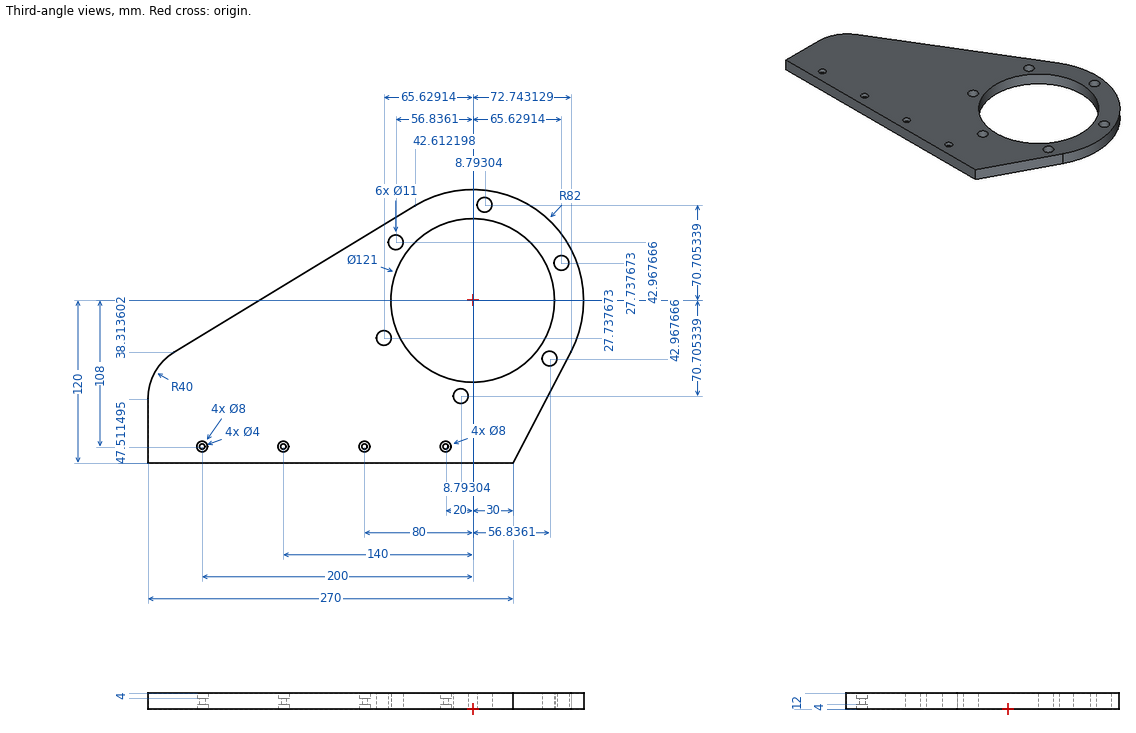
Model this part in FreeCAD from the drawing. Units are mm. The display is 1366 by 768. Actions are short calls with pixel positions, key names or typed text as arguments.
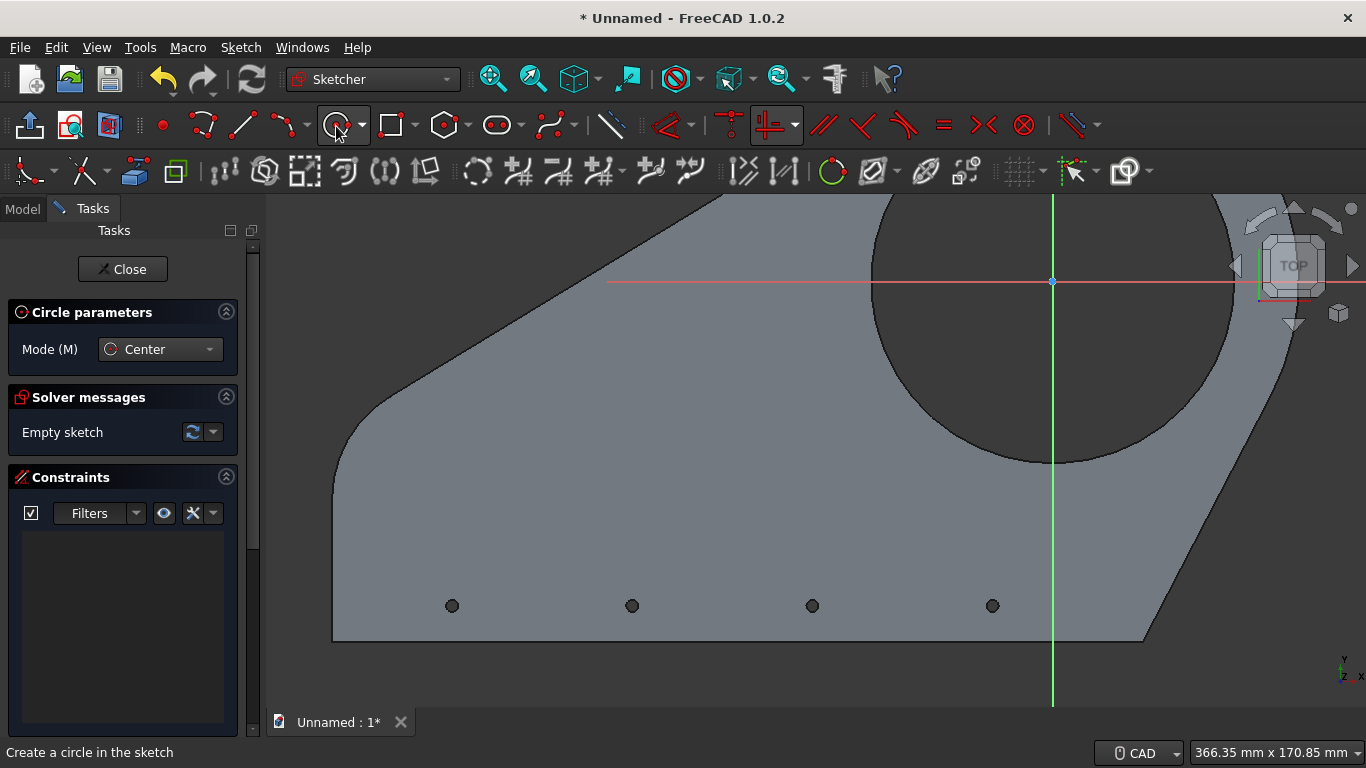
scroll(452, 606, up, 4)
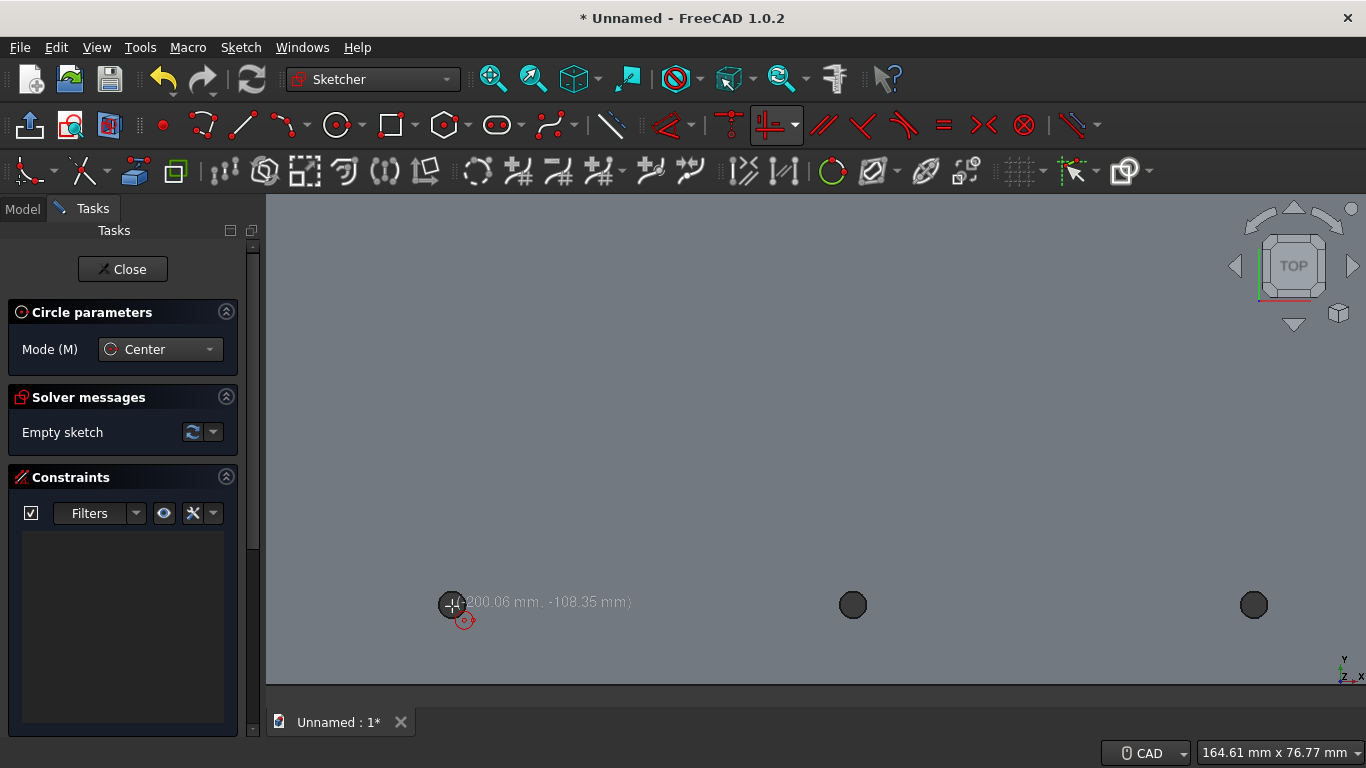
click(452, 605)
click(471, 586)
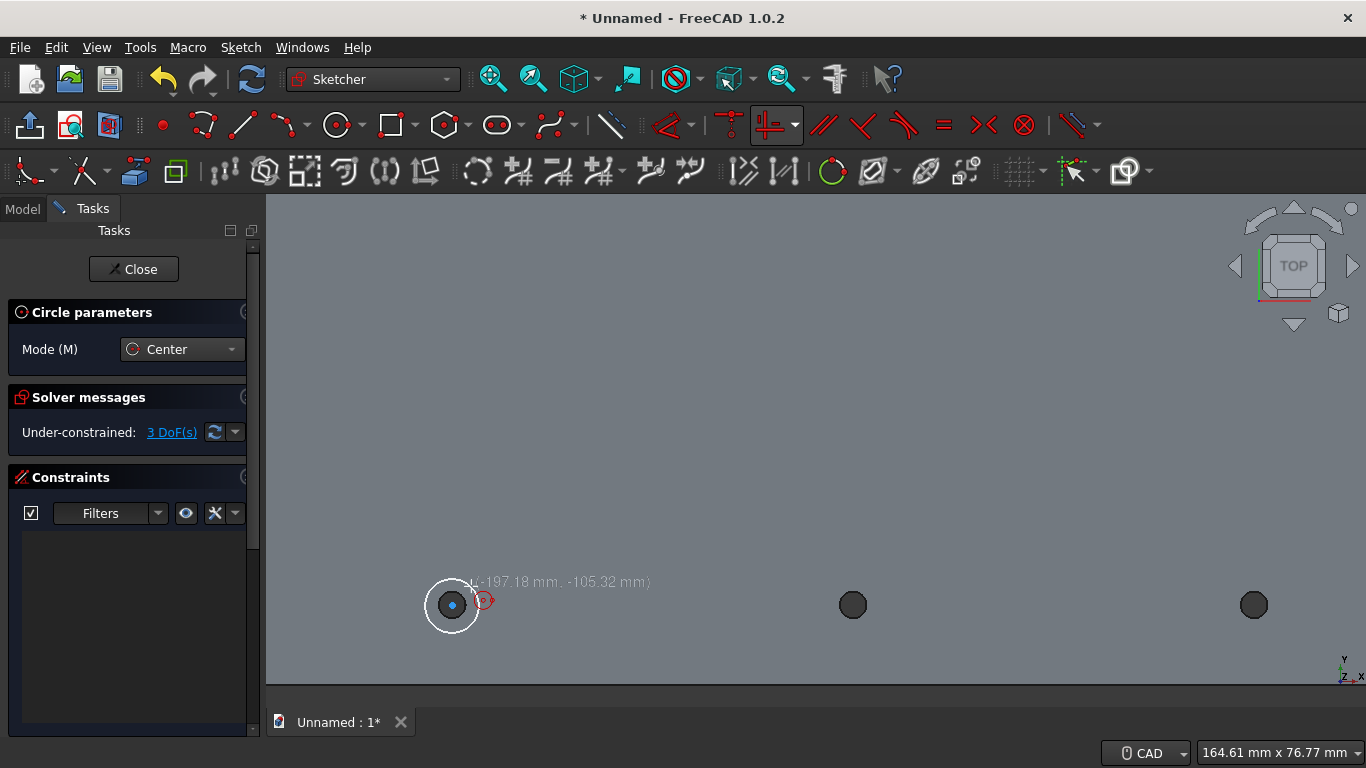
click(853, 605)
click(872, 586)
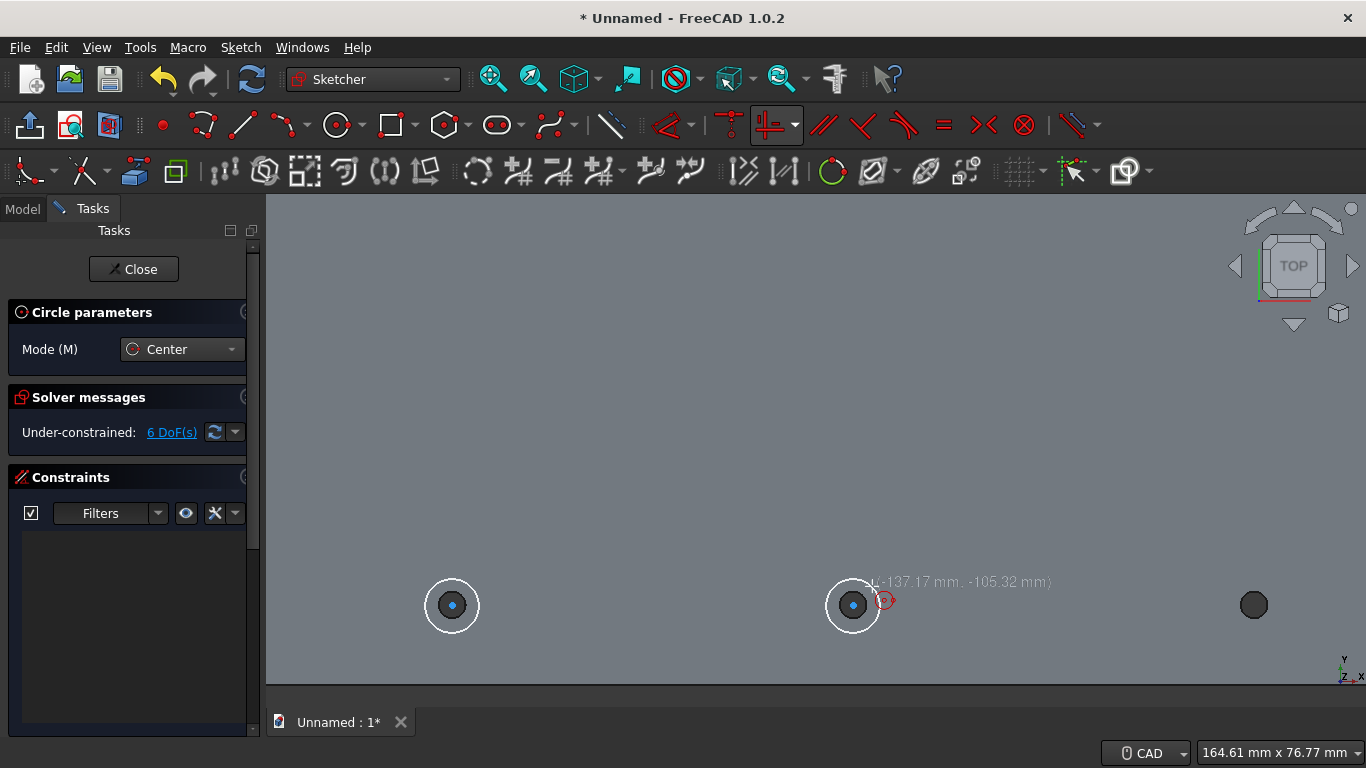
scroll(454, 608, down, 4)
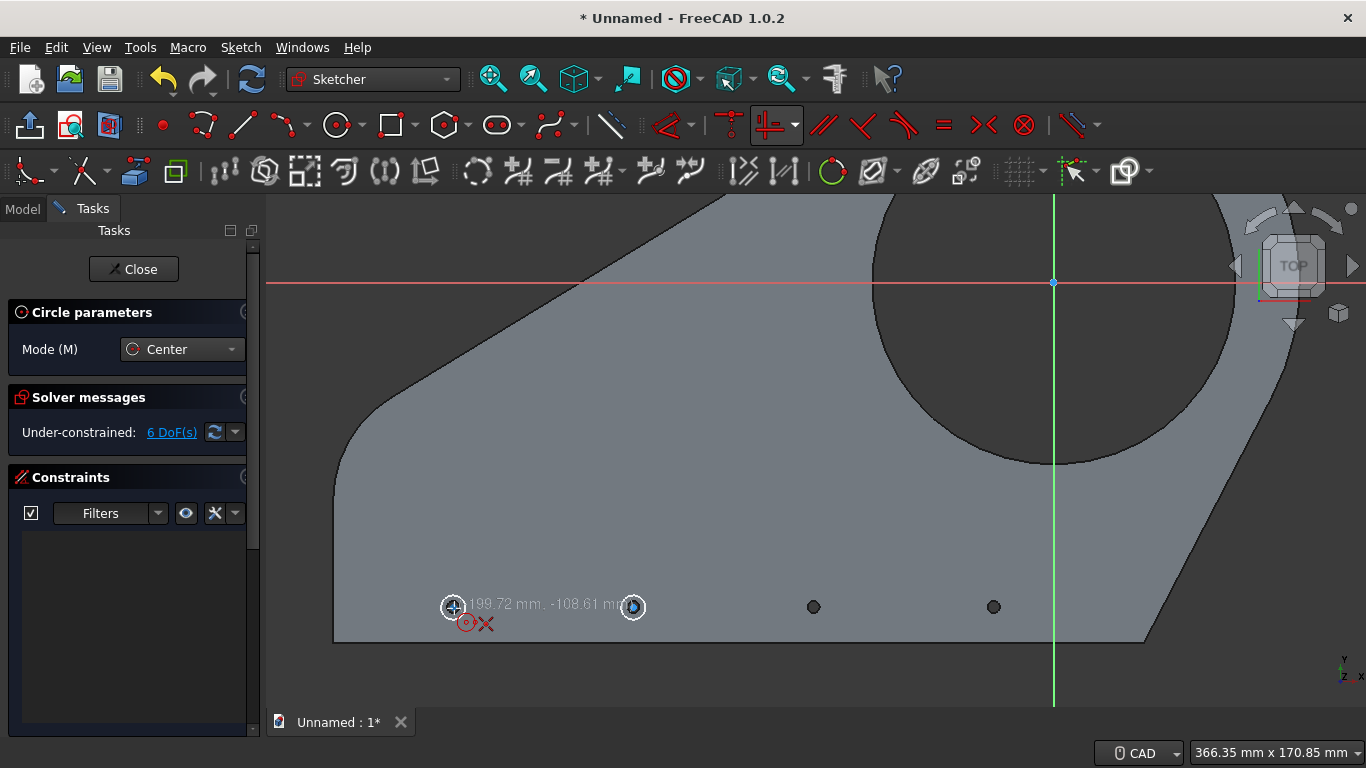
scroll(814, 607, up, 4)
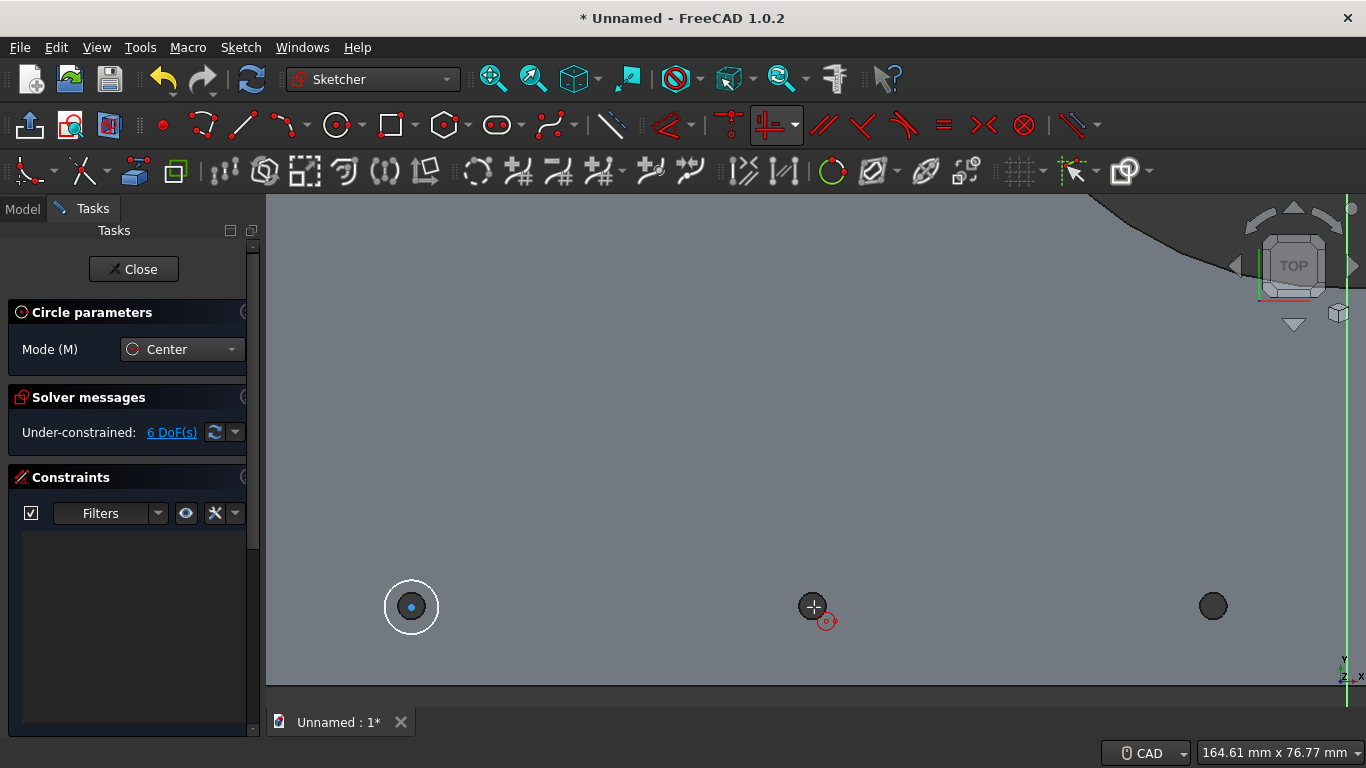
click(812, 606)
click(831, 587)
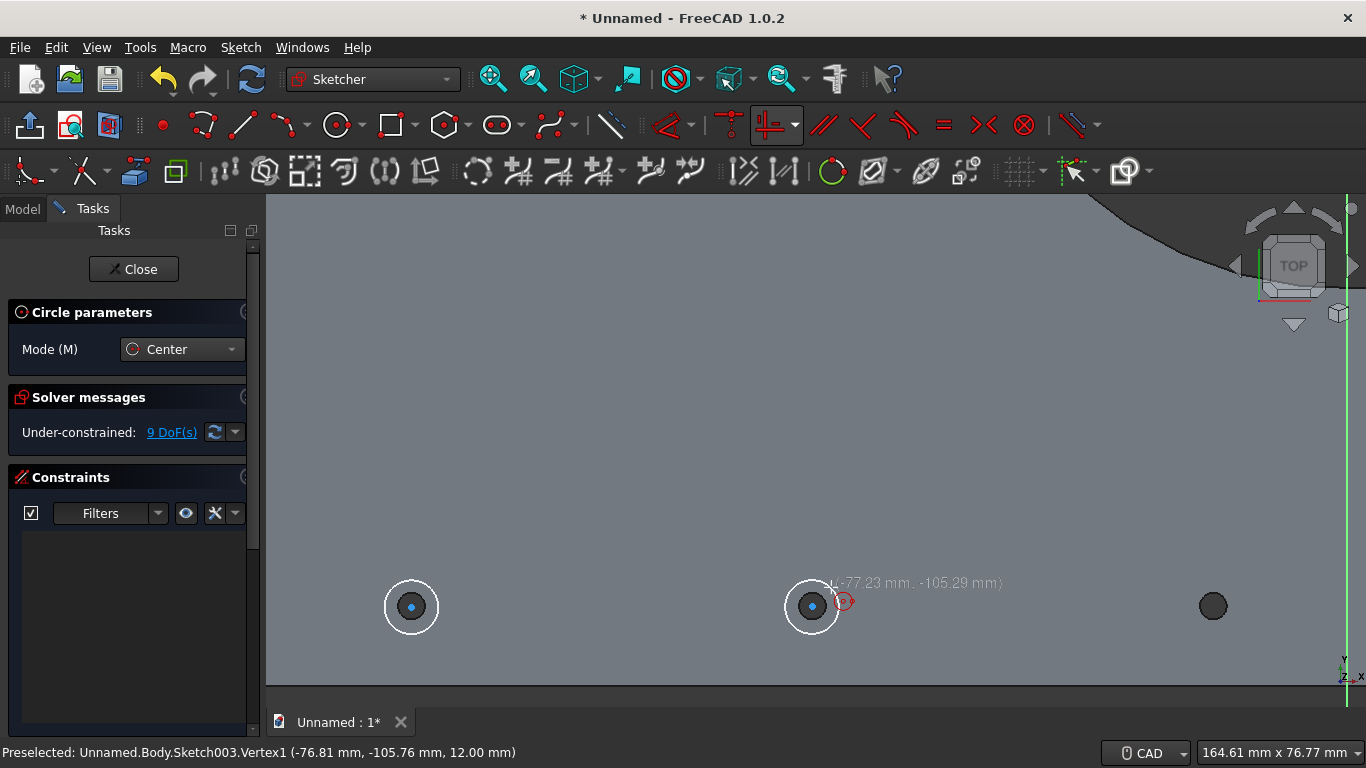
scroll(814, 607, down, 4)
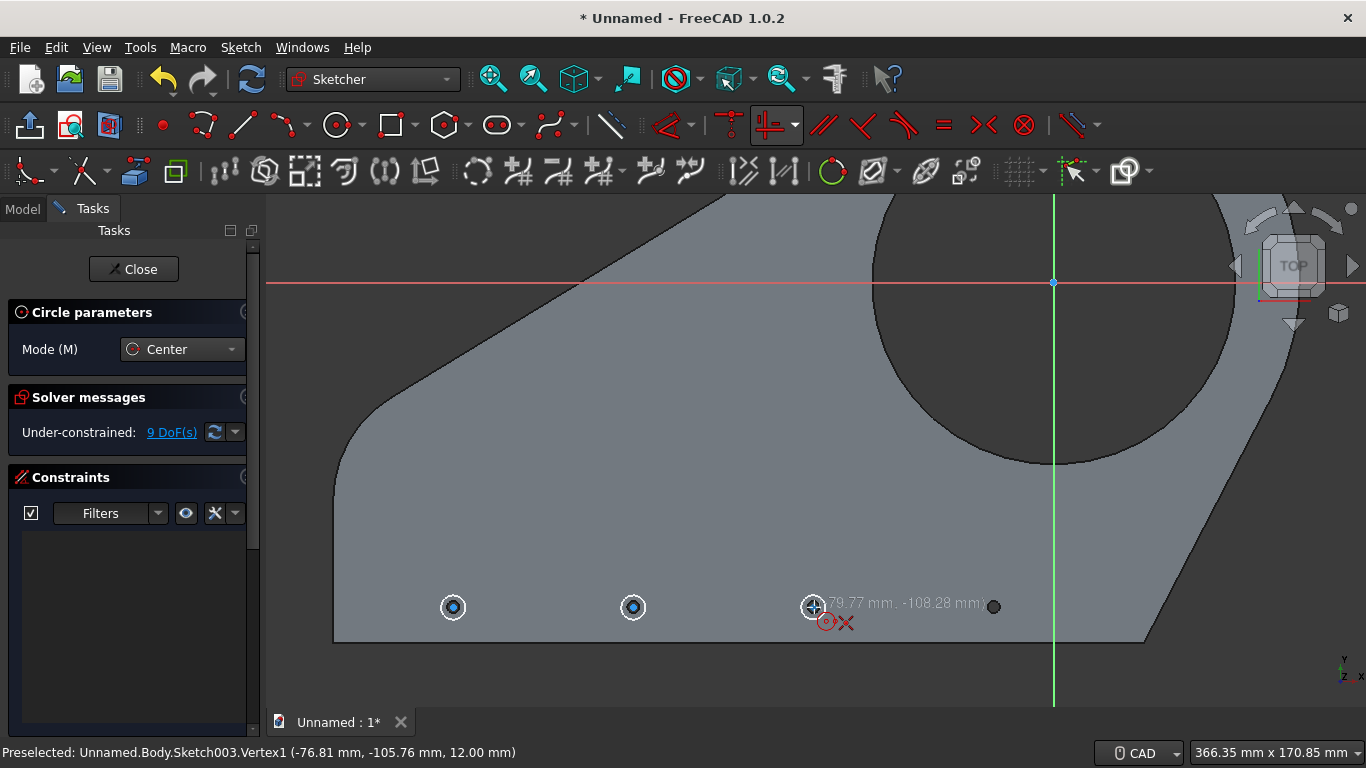
scroll(994, 607, up, 4)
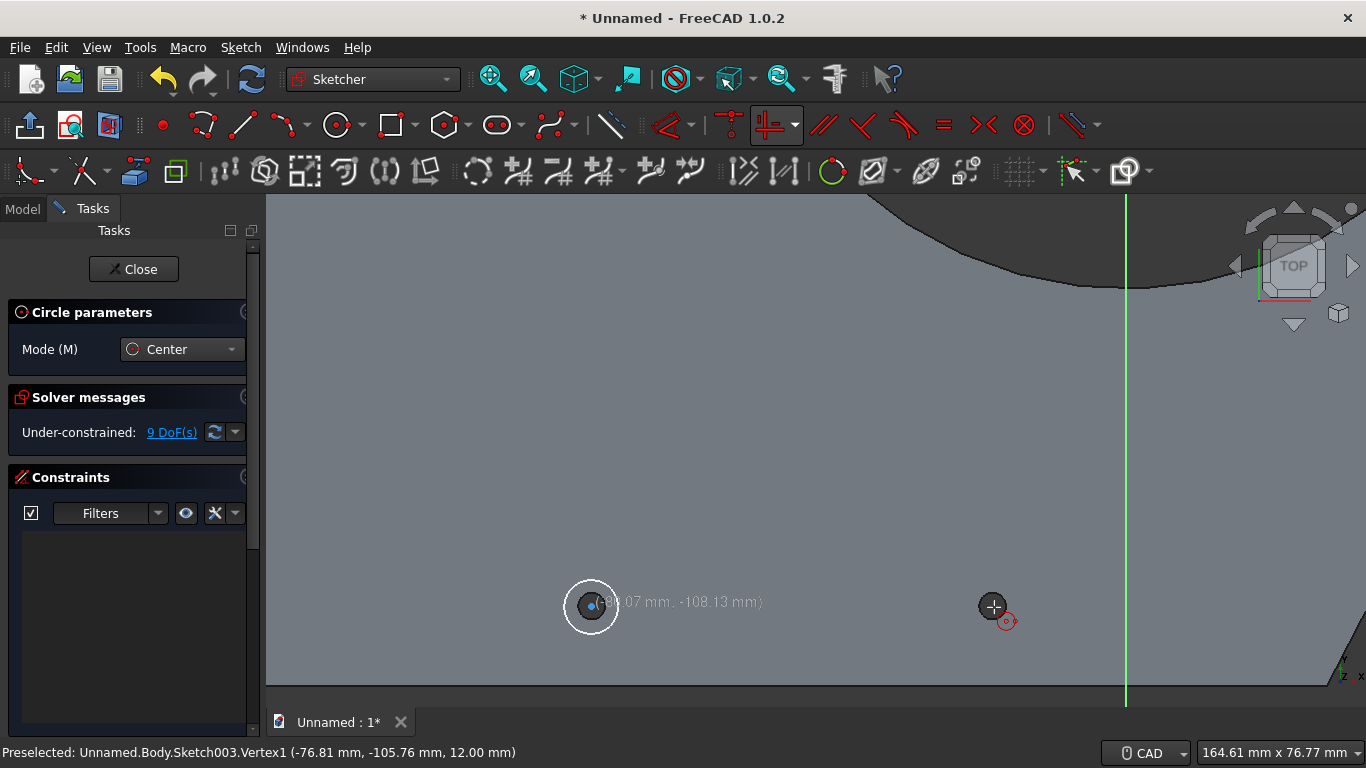
click(993, 606)
click(1012, 587)
key(Escape)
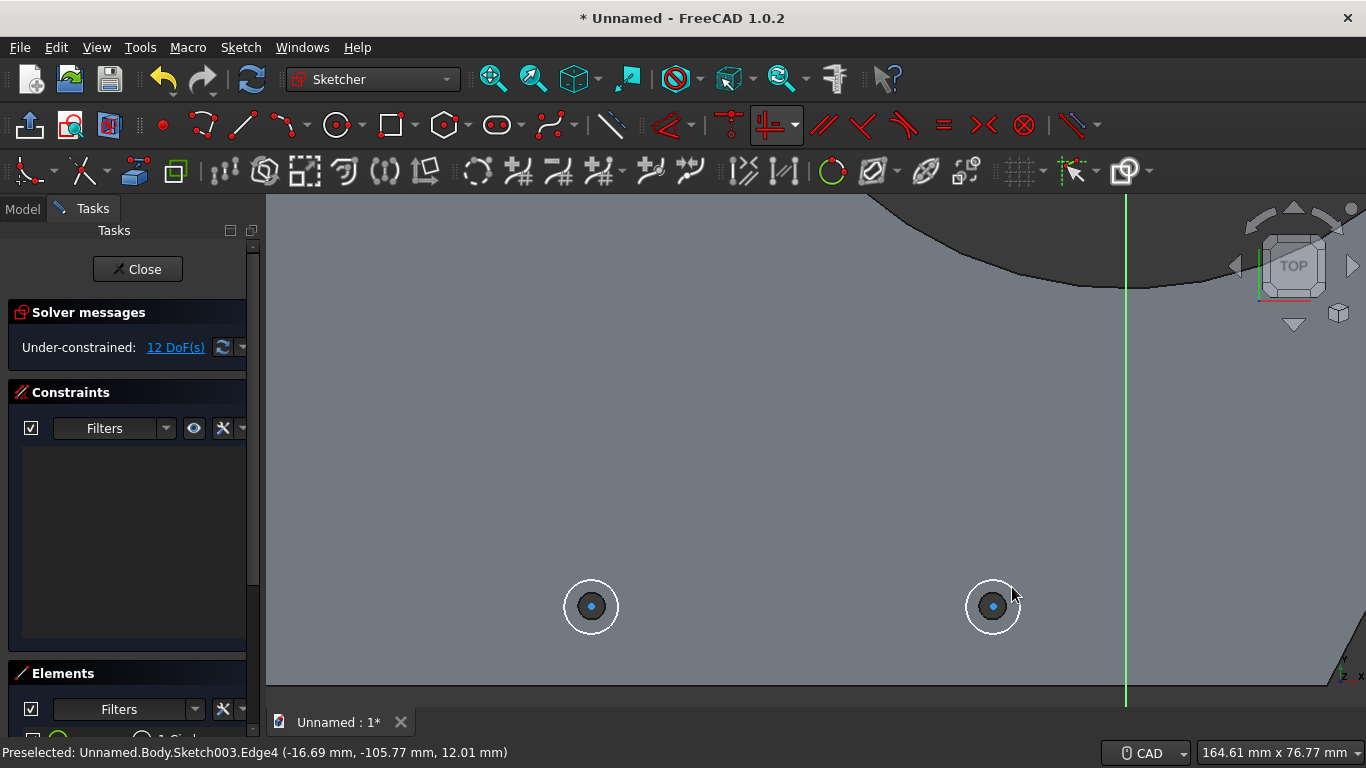
scroll(995, 607, down, 4)